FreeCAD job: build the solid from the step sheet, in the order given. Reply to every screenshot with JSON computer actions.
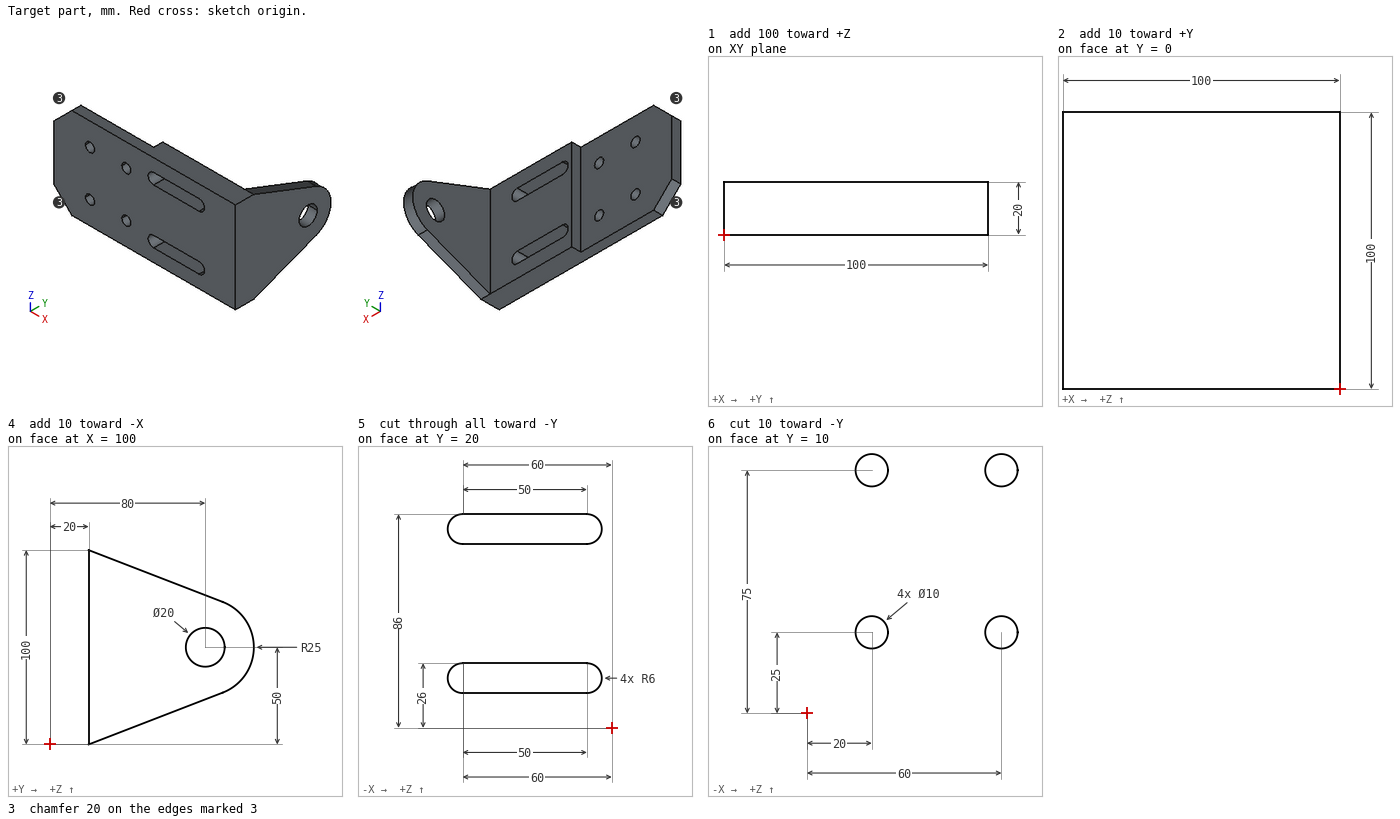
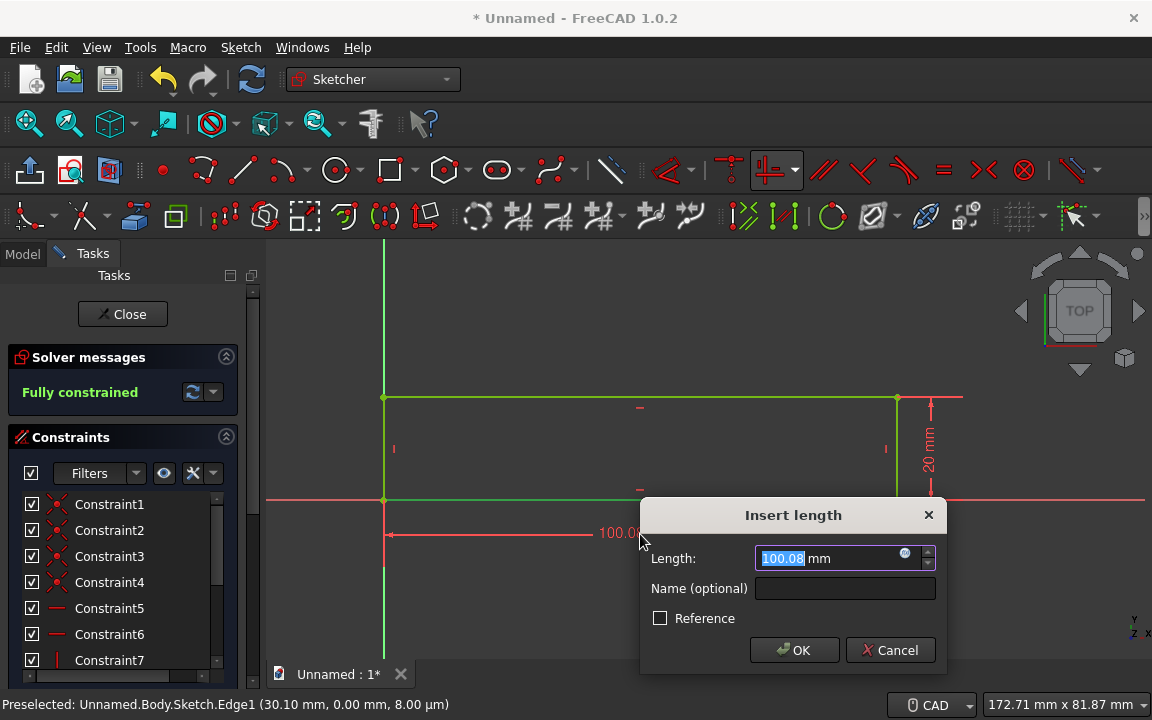
{"action": "type", "text": "100"}
{"action": "key", "text": "Return"}
{"action": "key", "text": "Escape"}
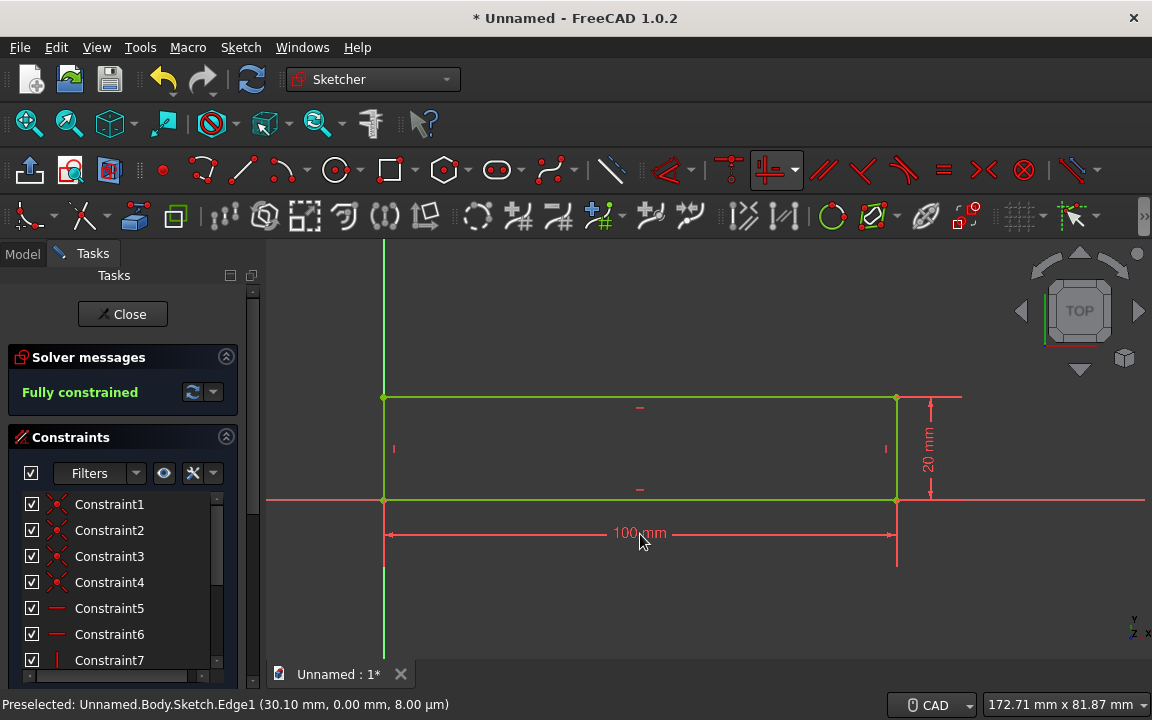
{"action": "left_click", "coordinate": [123, 314]}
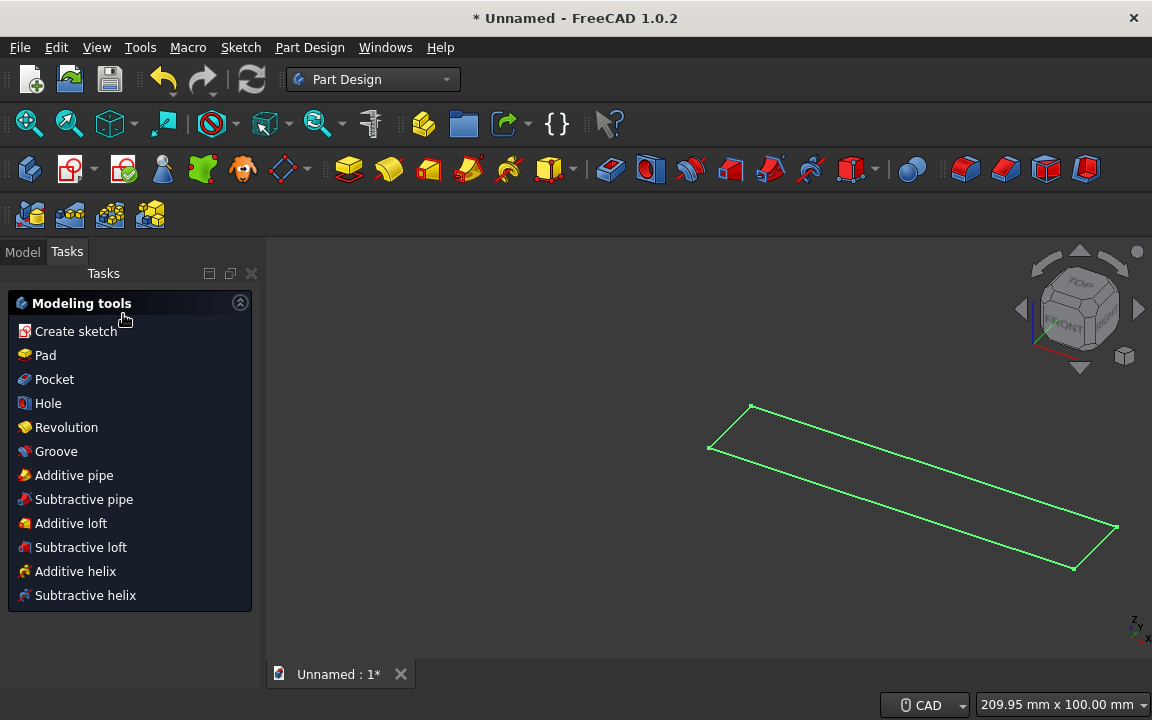
{"action": "left_click", "coordinate": [350, 170]}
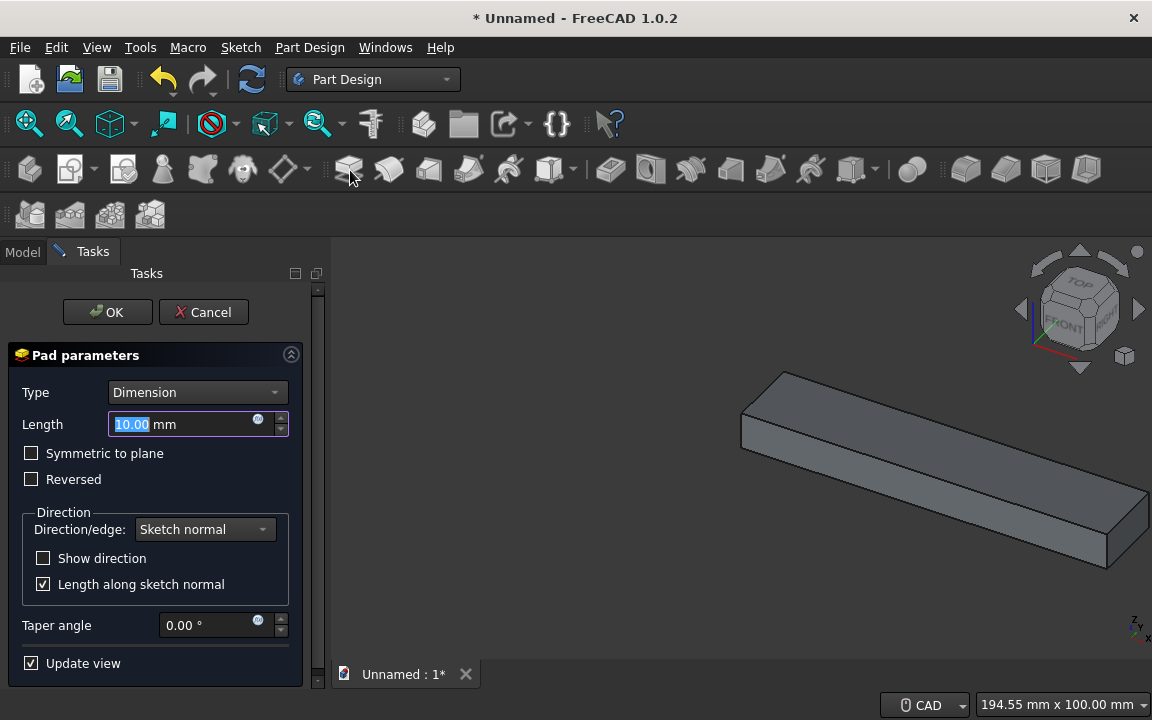
{"action": "type", "text": "100"}
{"action": "key", "text": "Tab"}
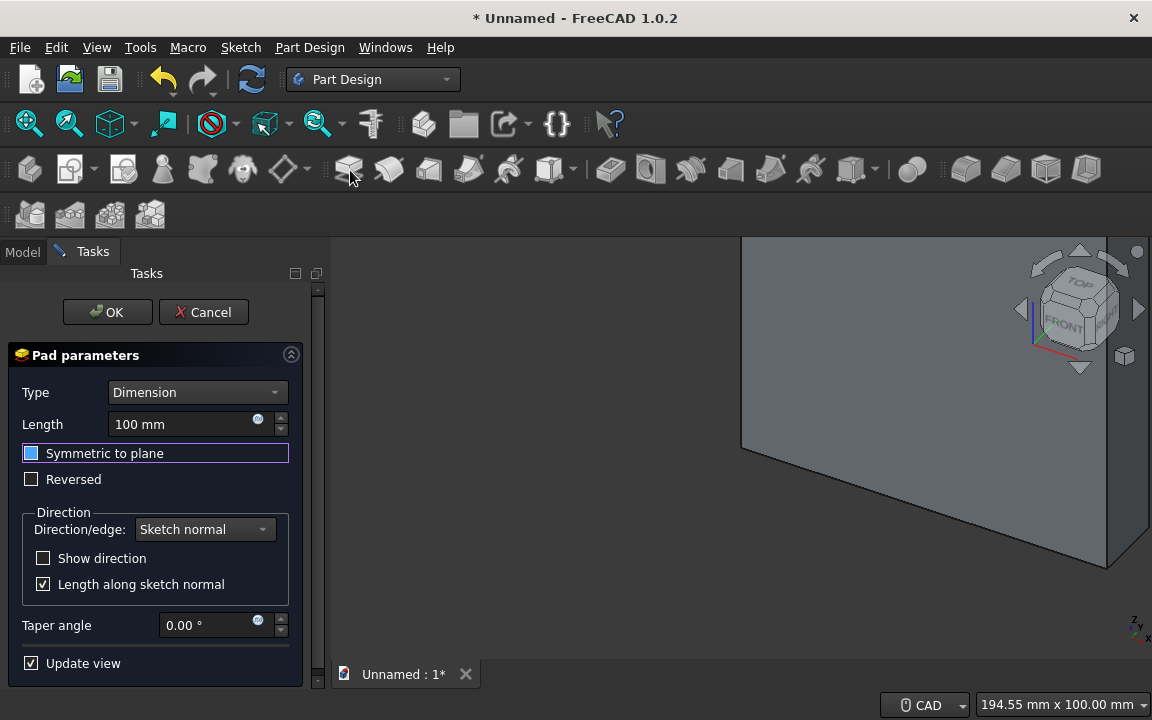
{"action": "left_click", "coordinate": [108, 312]}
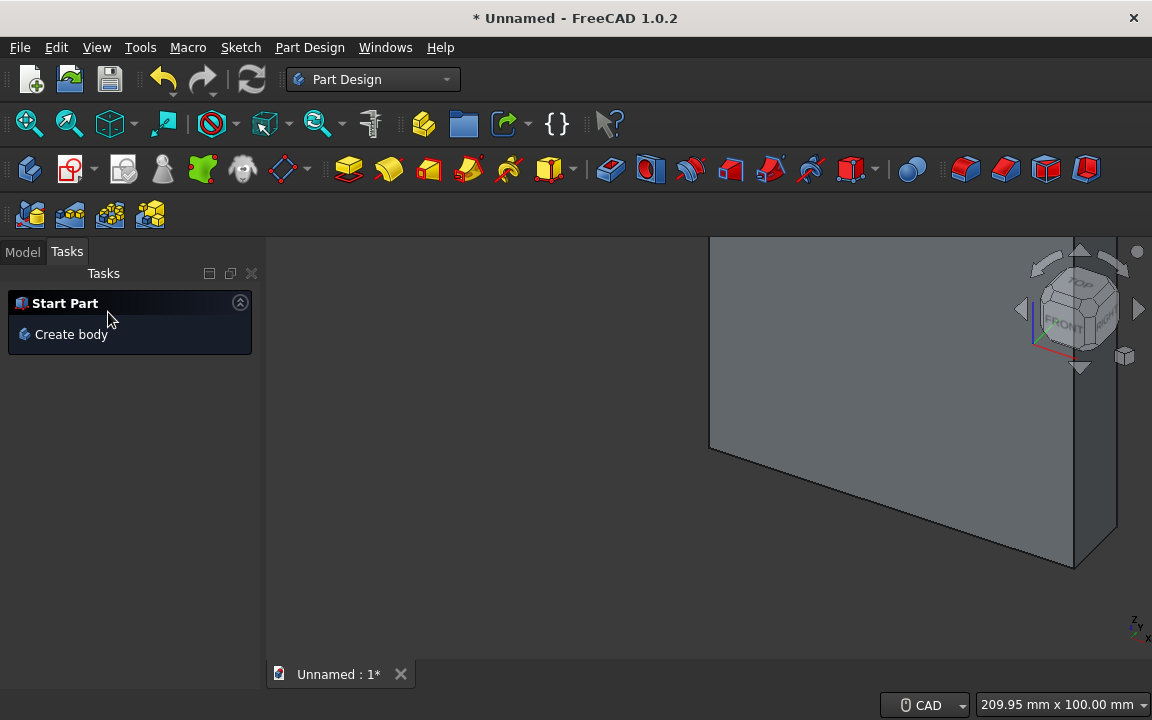
{"action": "left_click", "coordinate": [30, 124]}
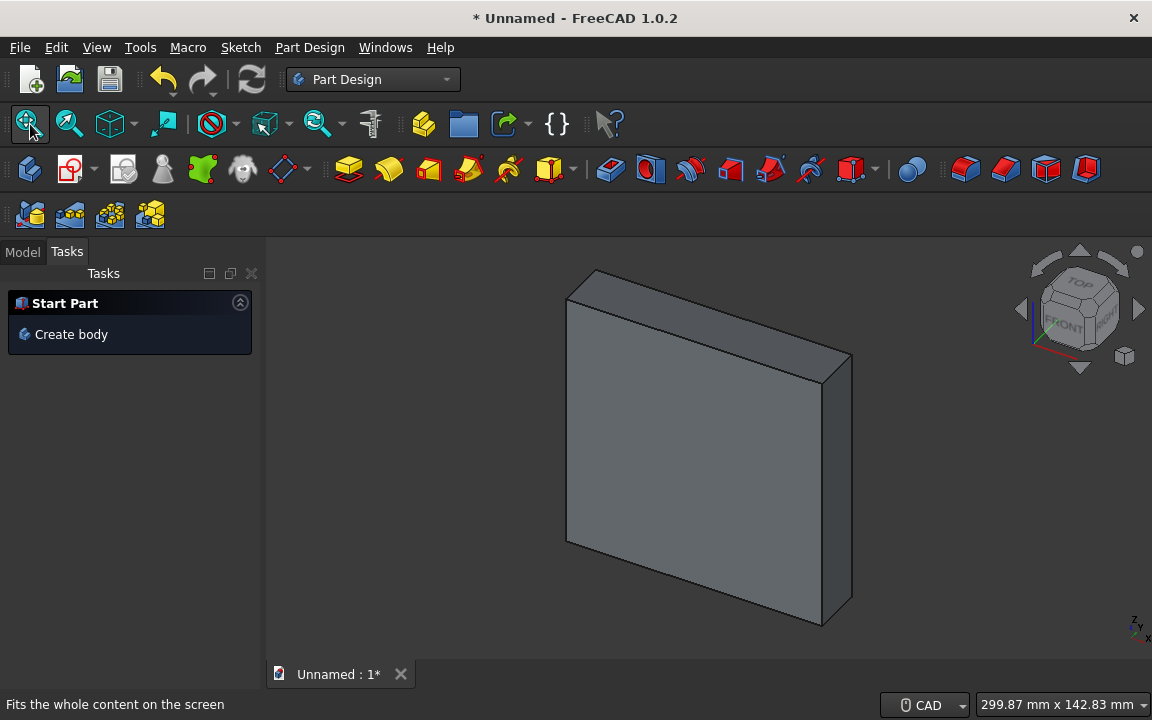
{"action": "left_click", "coordinate": [694, 462]}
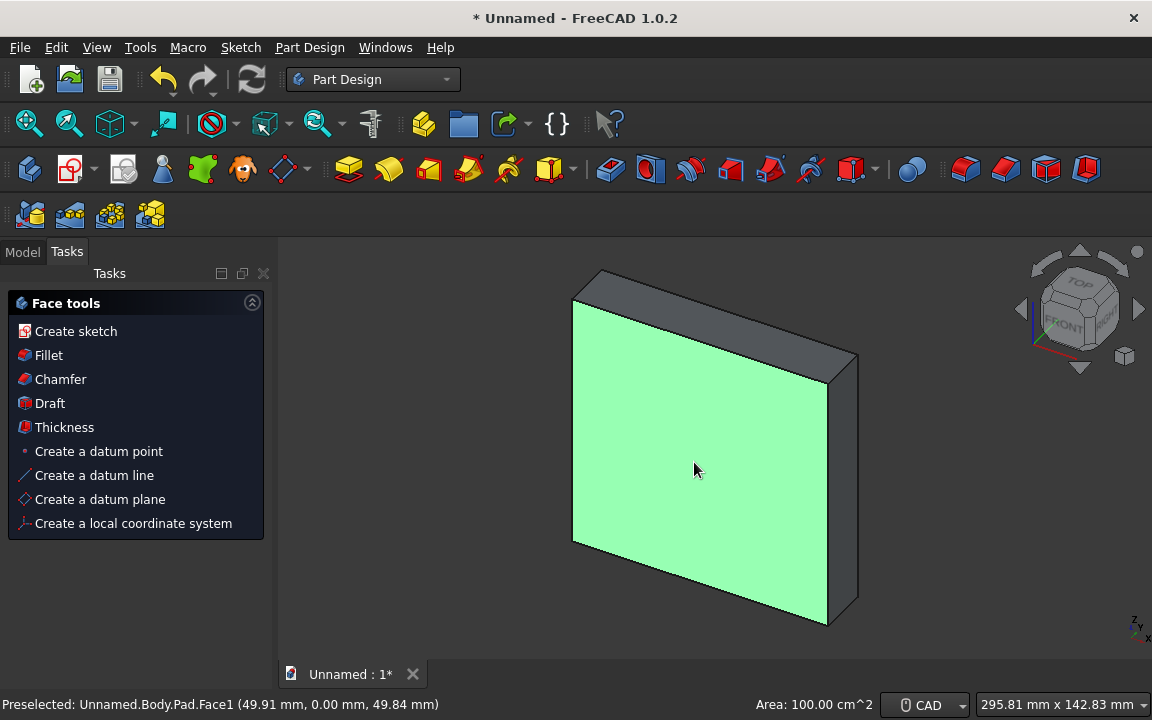
{"action": "left_click", "coordinate": [70, 170]}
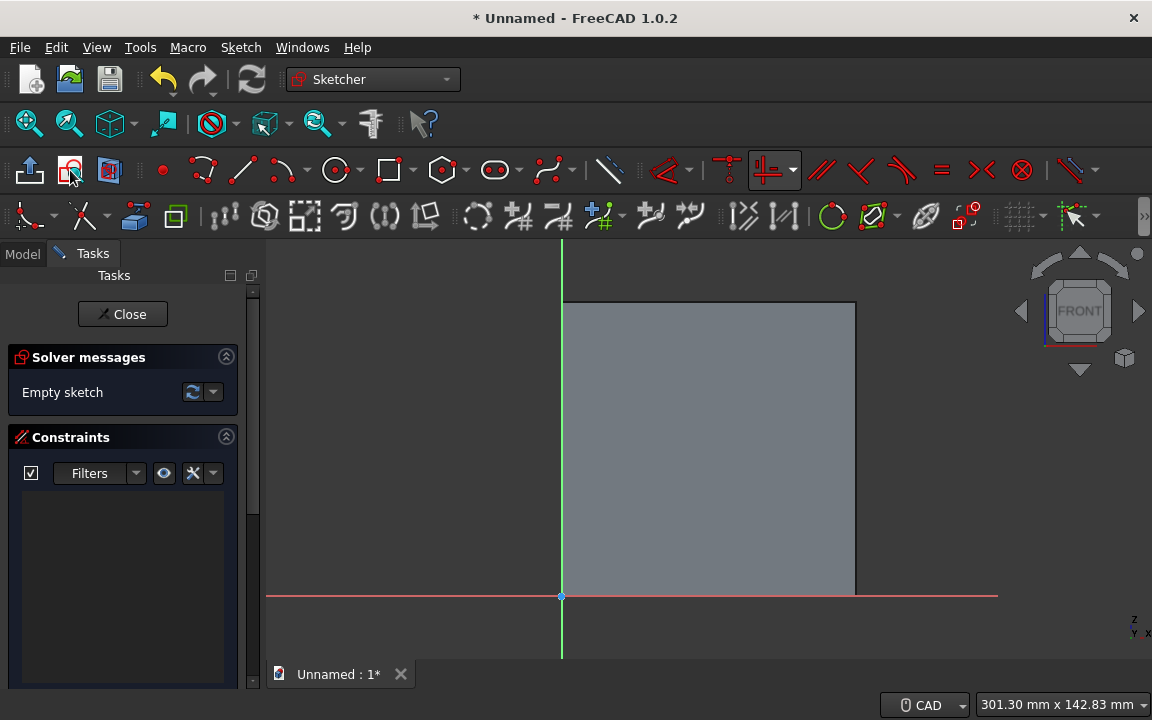
{"action": "scroll", "coordinate": [987, 449], "scroll_direction": "down", "scroll_amount": 1}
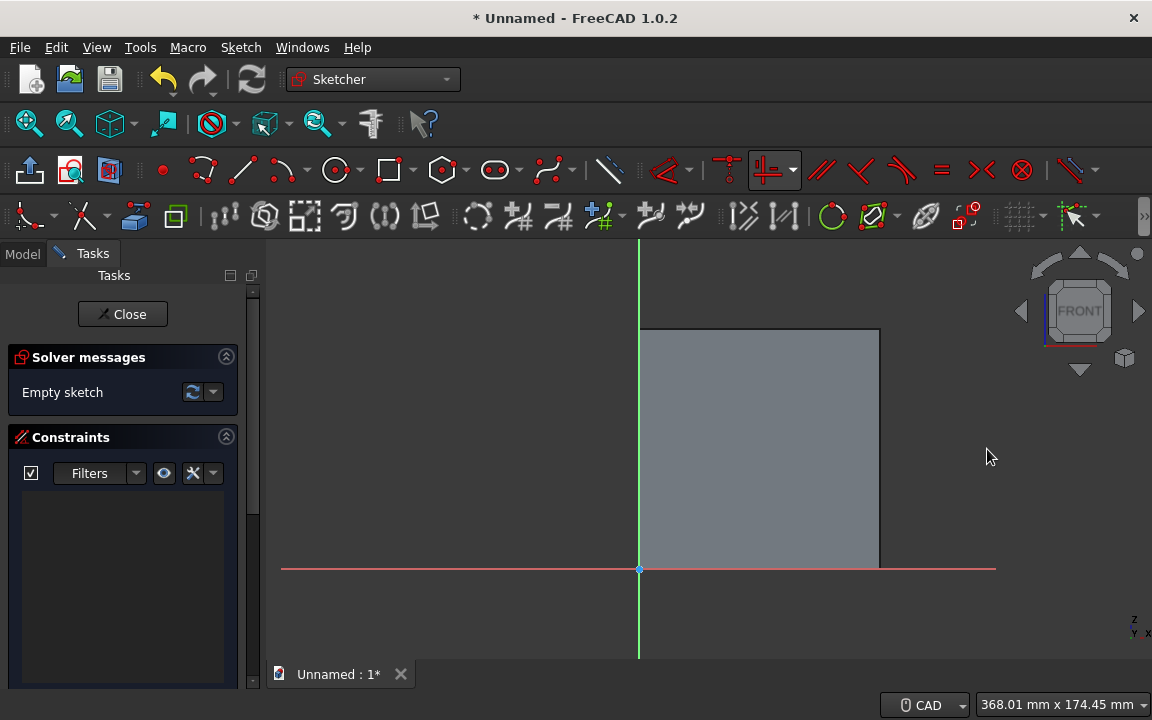
{"action": "left_click", "coordinate": [390, 170]}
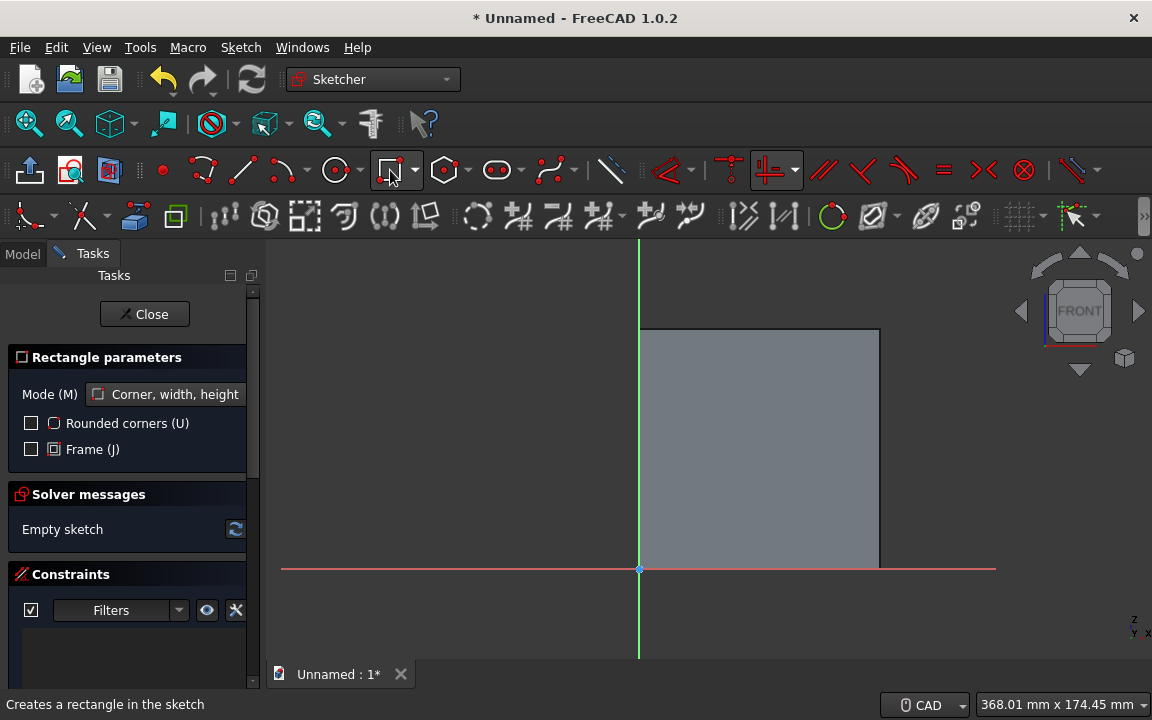
{"action": "left_click", "coordinate": [639, 569]}
{"action": "left_click", "coordinate": [398, 329]}
{"action": "key", "text": "Escape"}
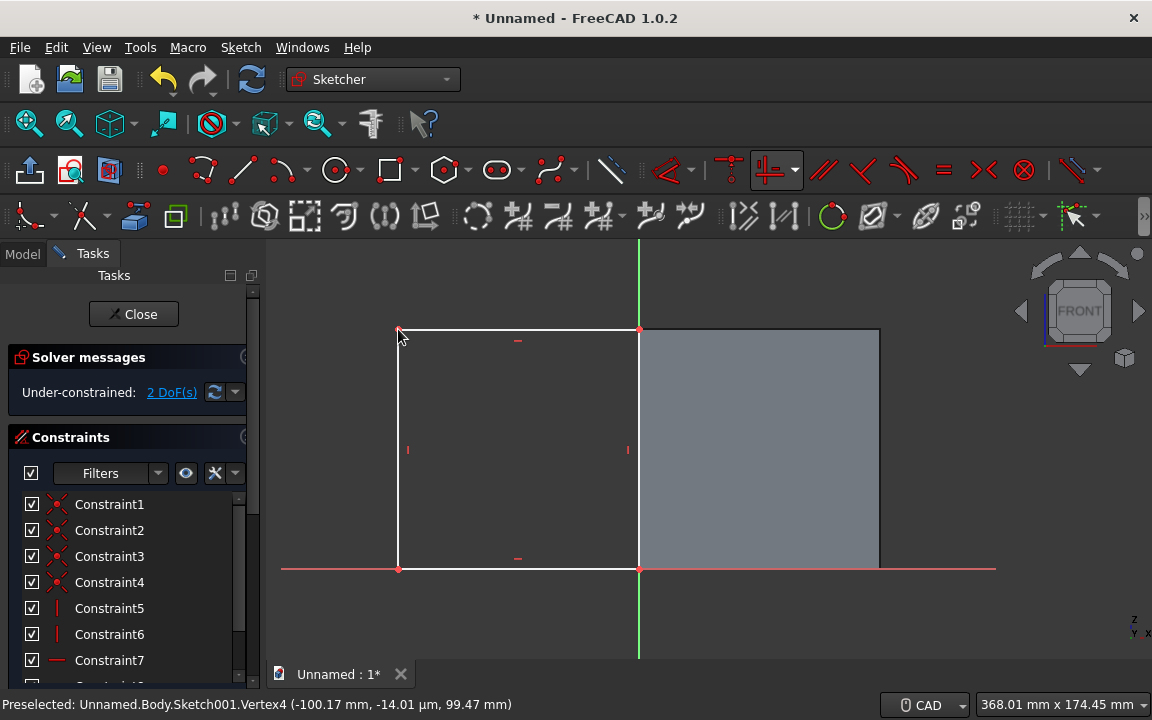
{"action": "left_click", "coordinate": [666, 170]}